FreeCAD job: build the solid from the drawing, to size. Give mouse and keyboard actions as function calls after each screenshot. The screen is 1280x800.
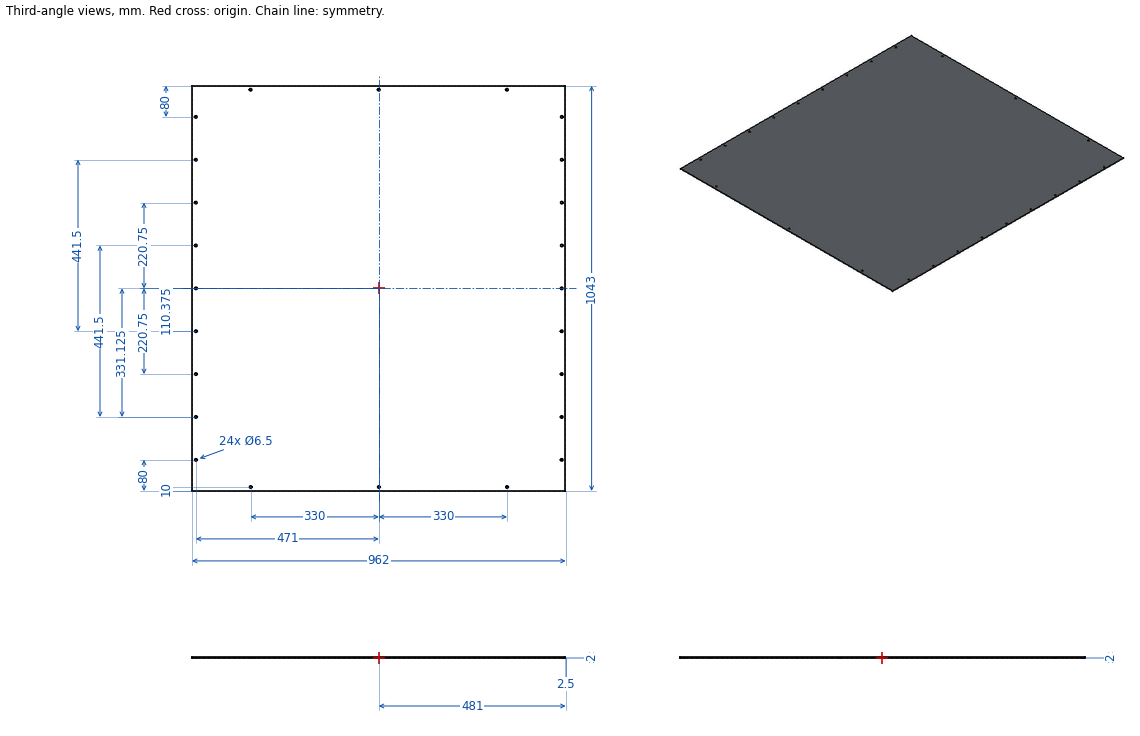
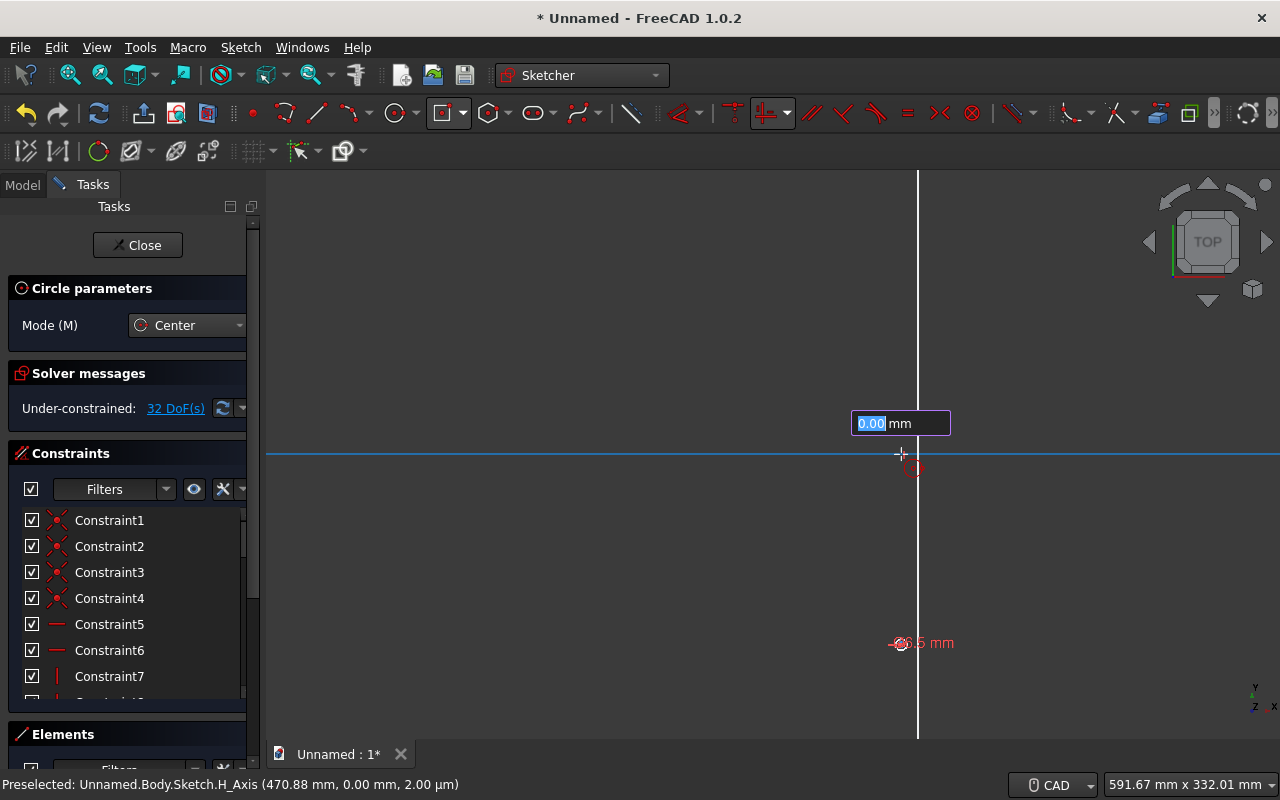
scroll(899, 460, up, 6)
move(899, 458)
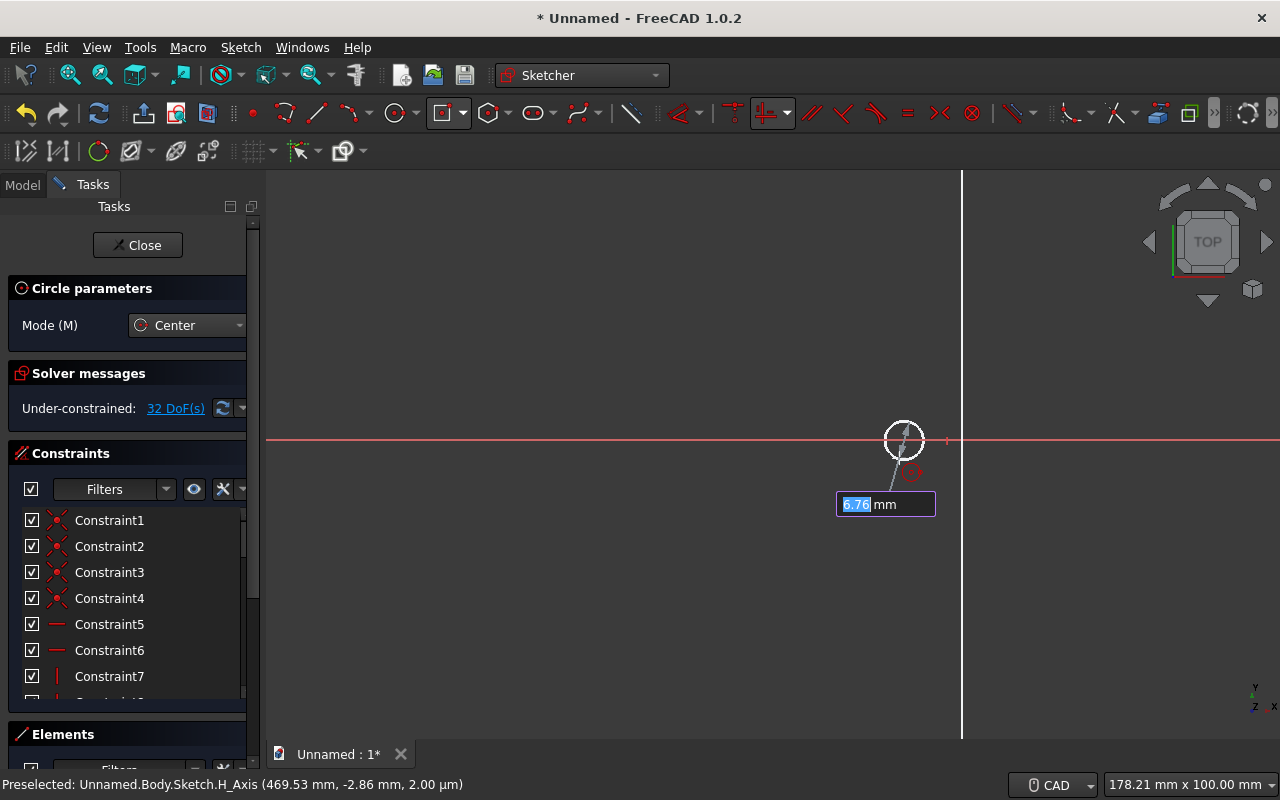
text(6.5)
key(Return)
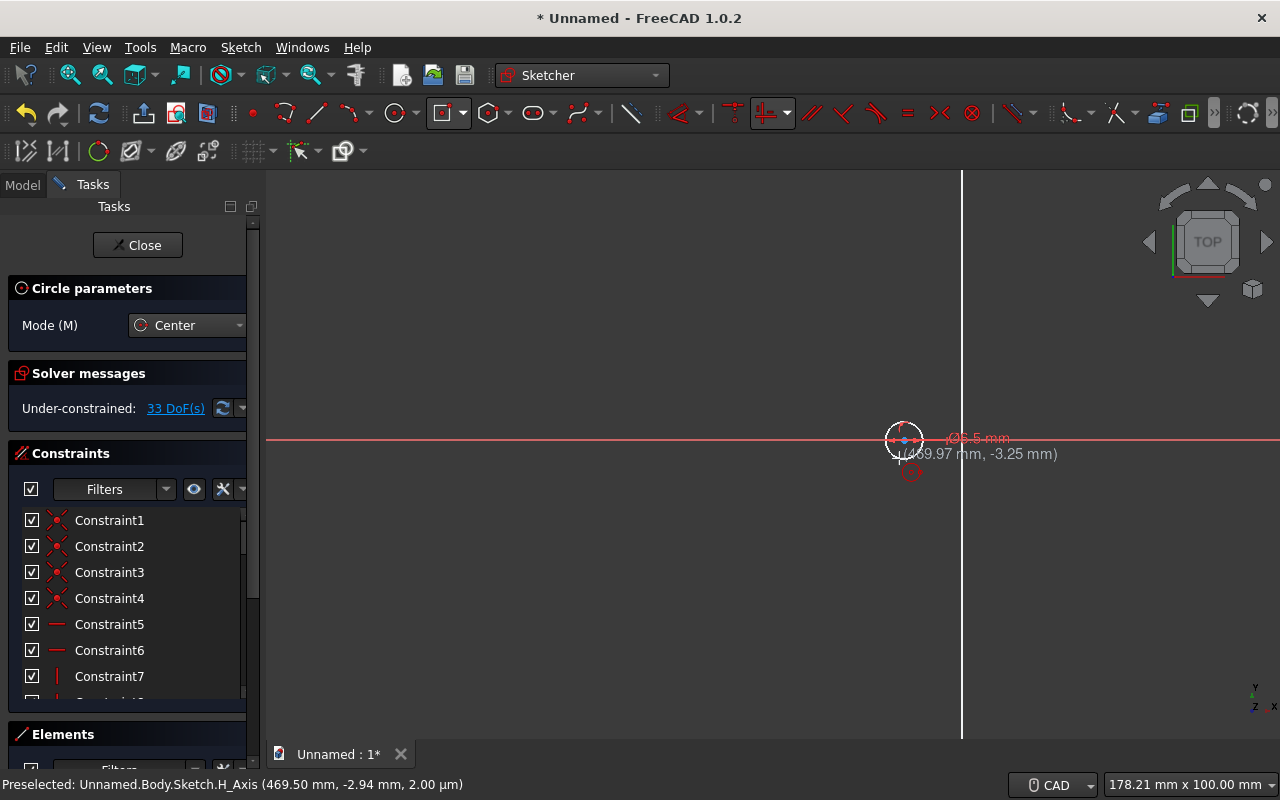
scroll(865, 455, down, 14)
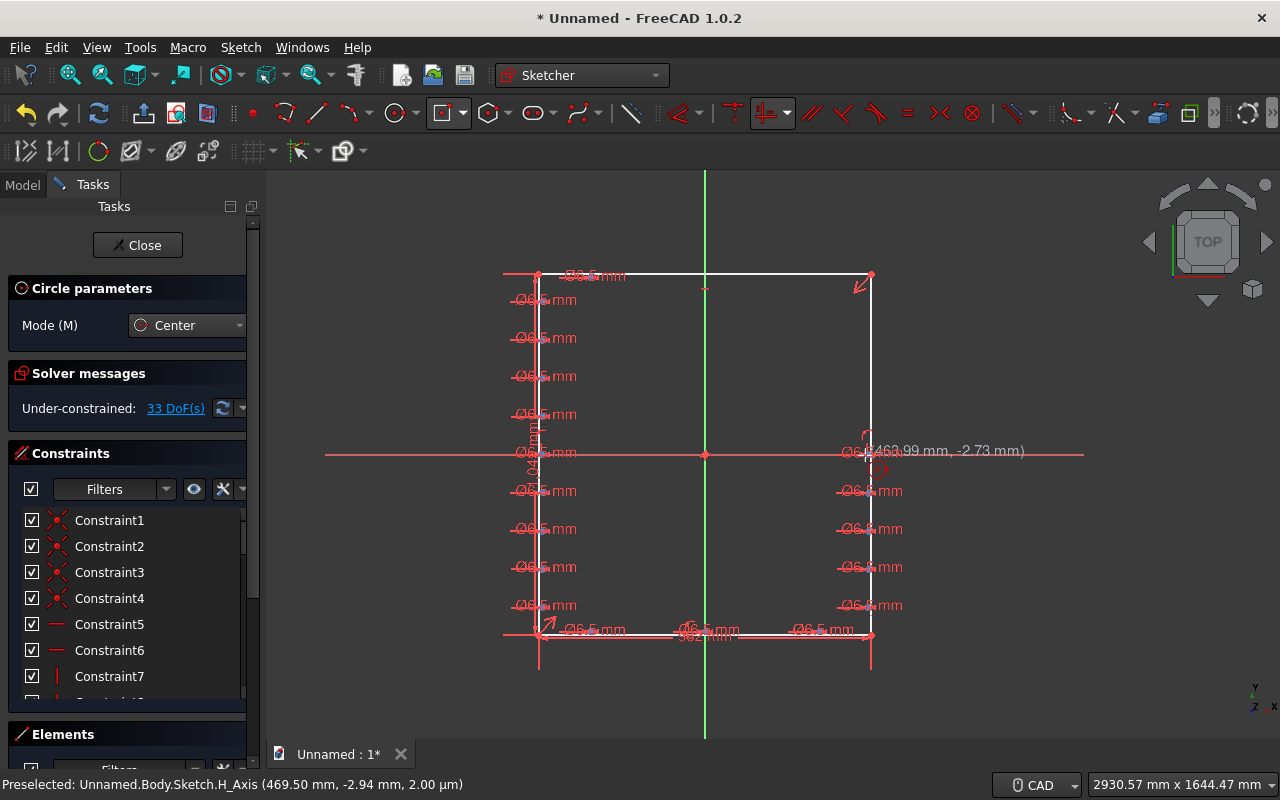
scroll(868, 416, up, 16)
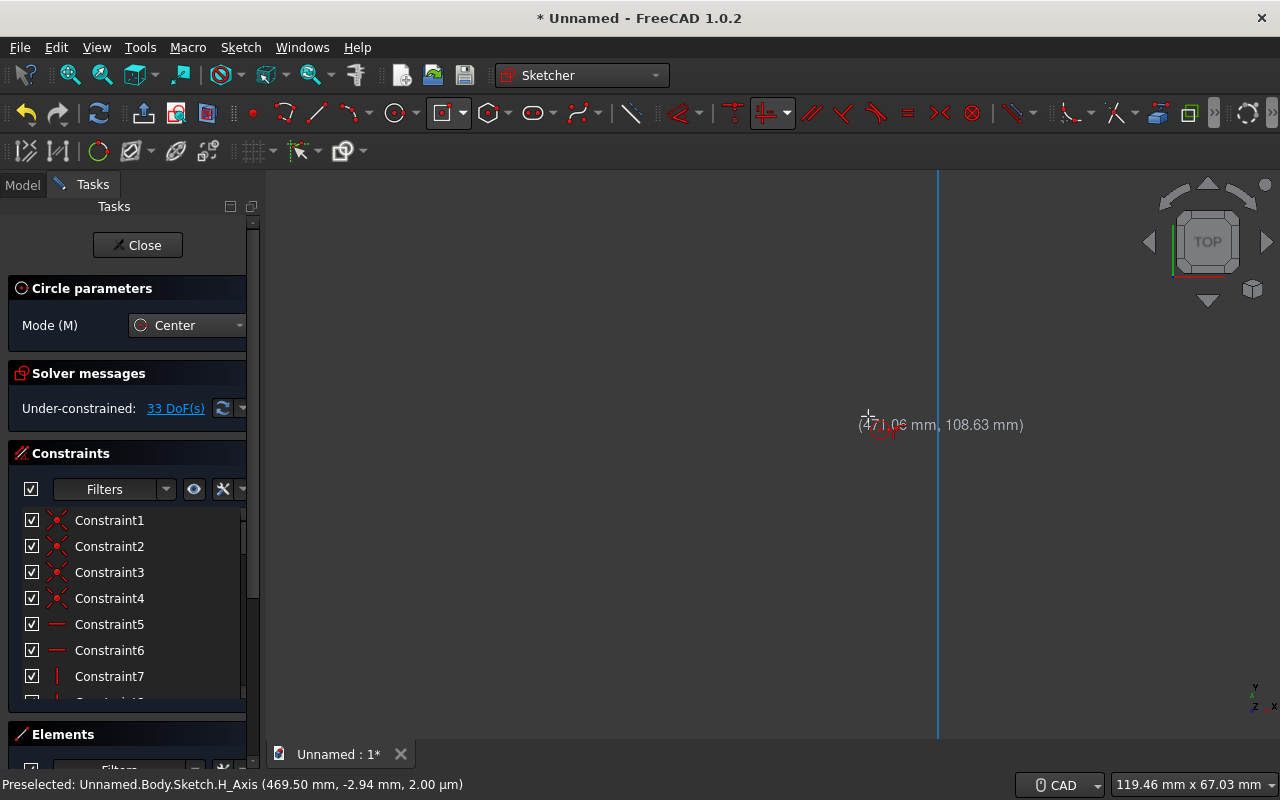
scroll(906, 407, down, 15)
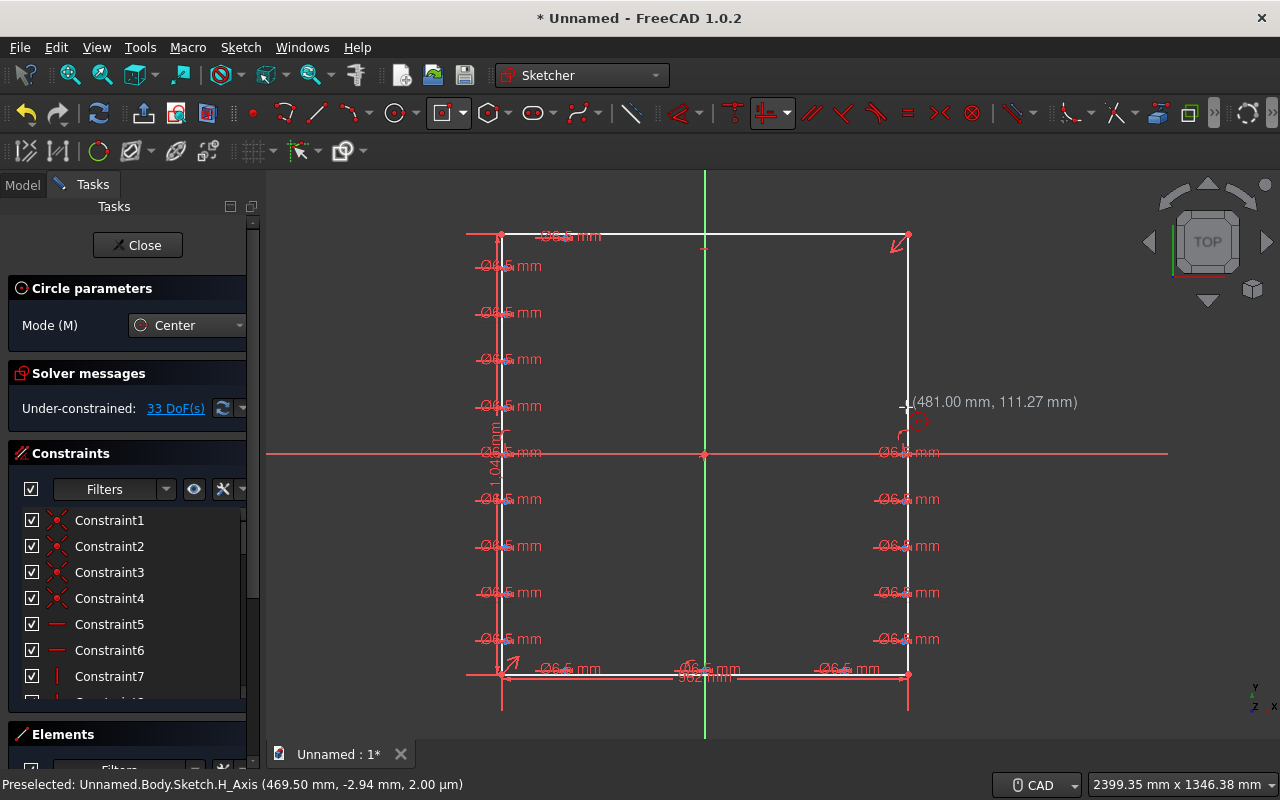
scroll(904, 408, up, 7)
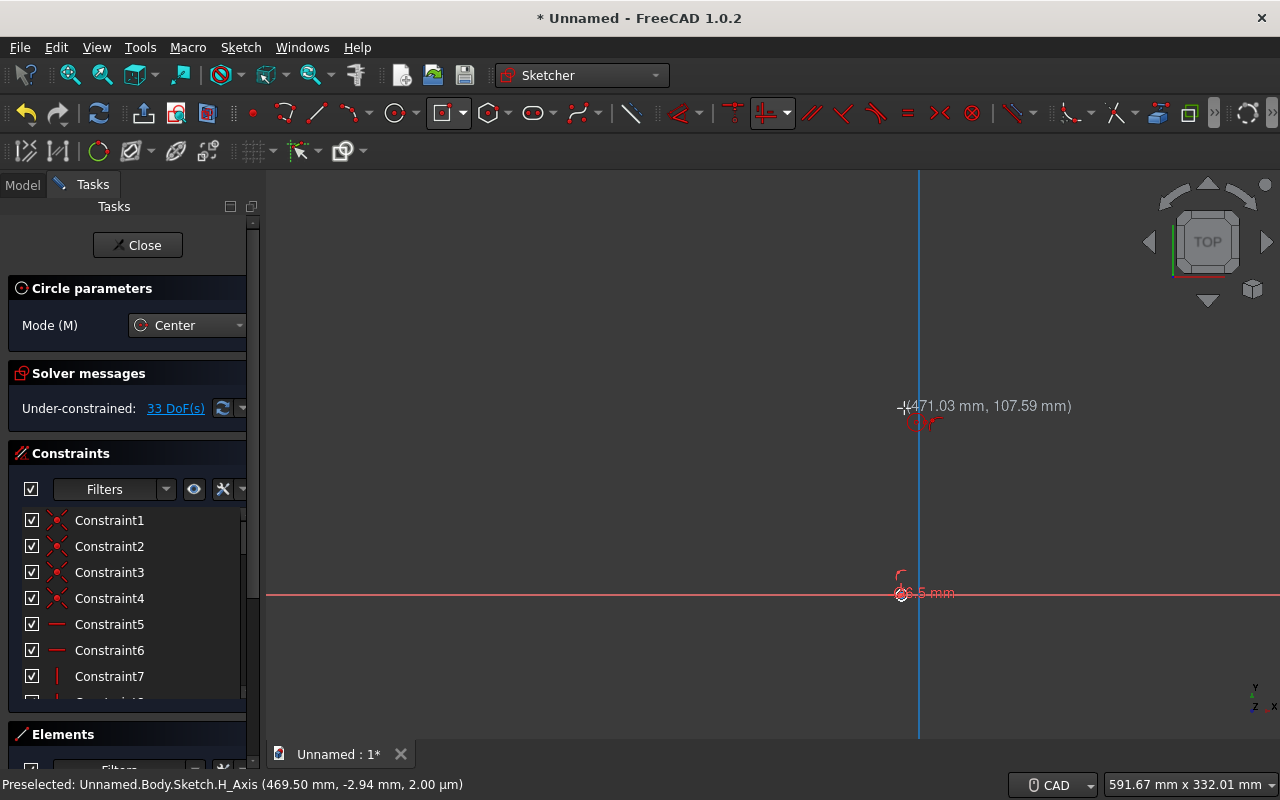
click(902, 406)
move(898, 402)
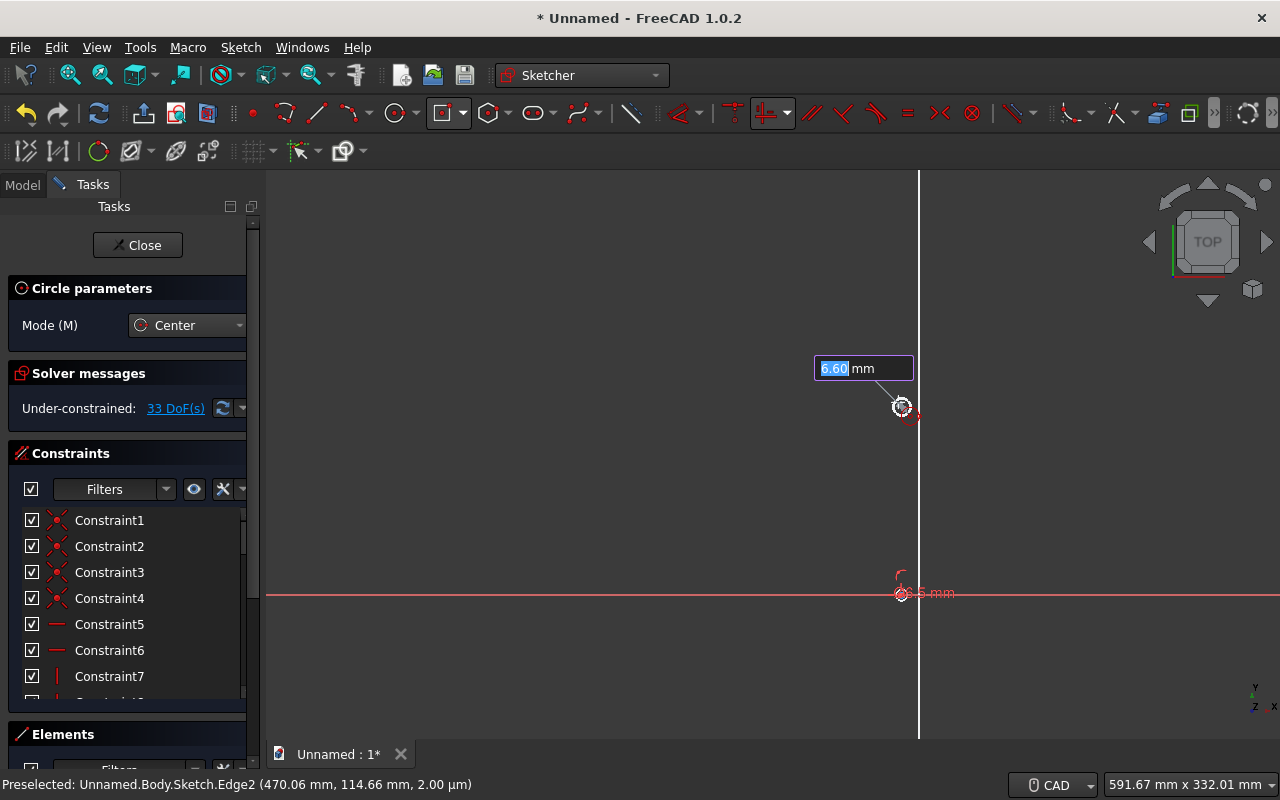
text(6.5)
key(Return)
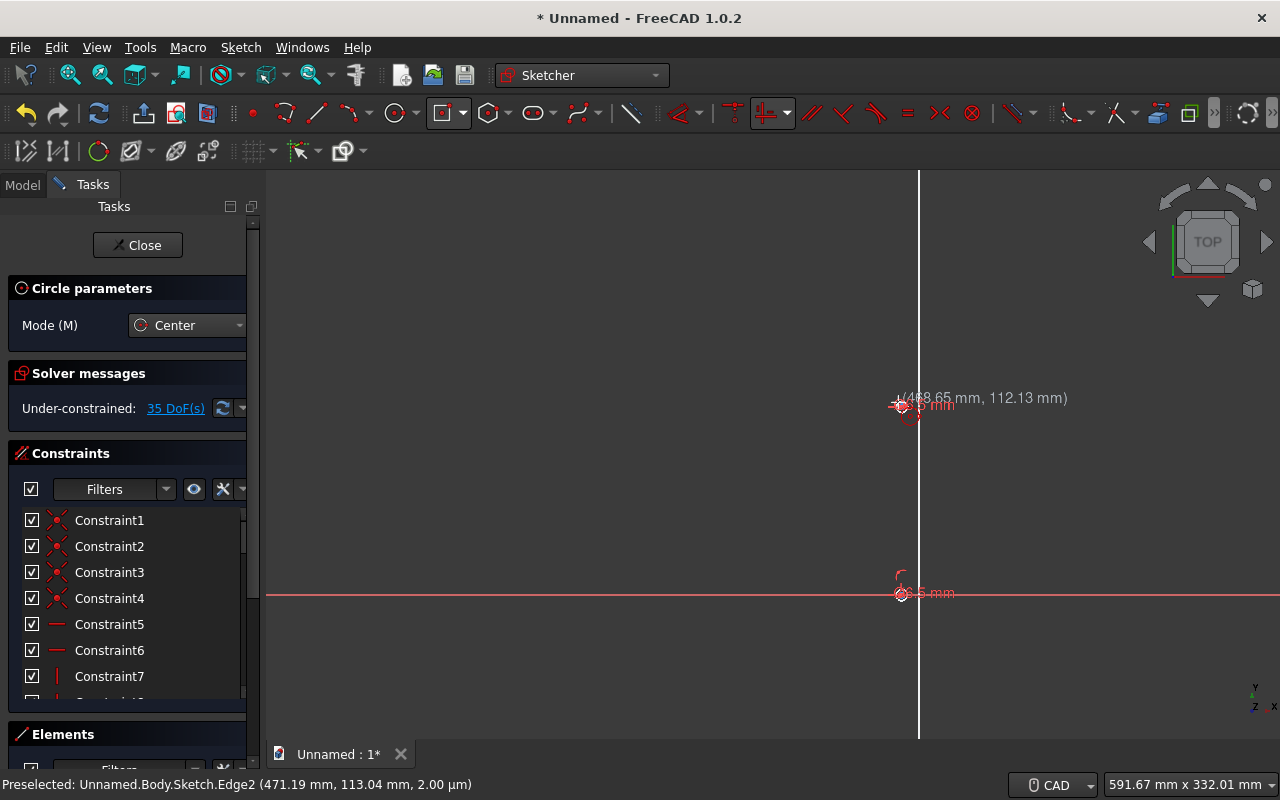
scroll(902, 217, up, 8)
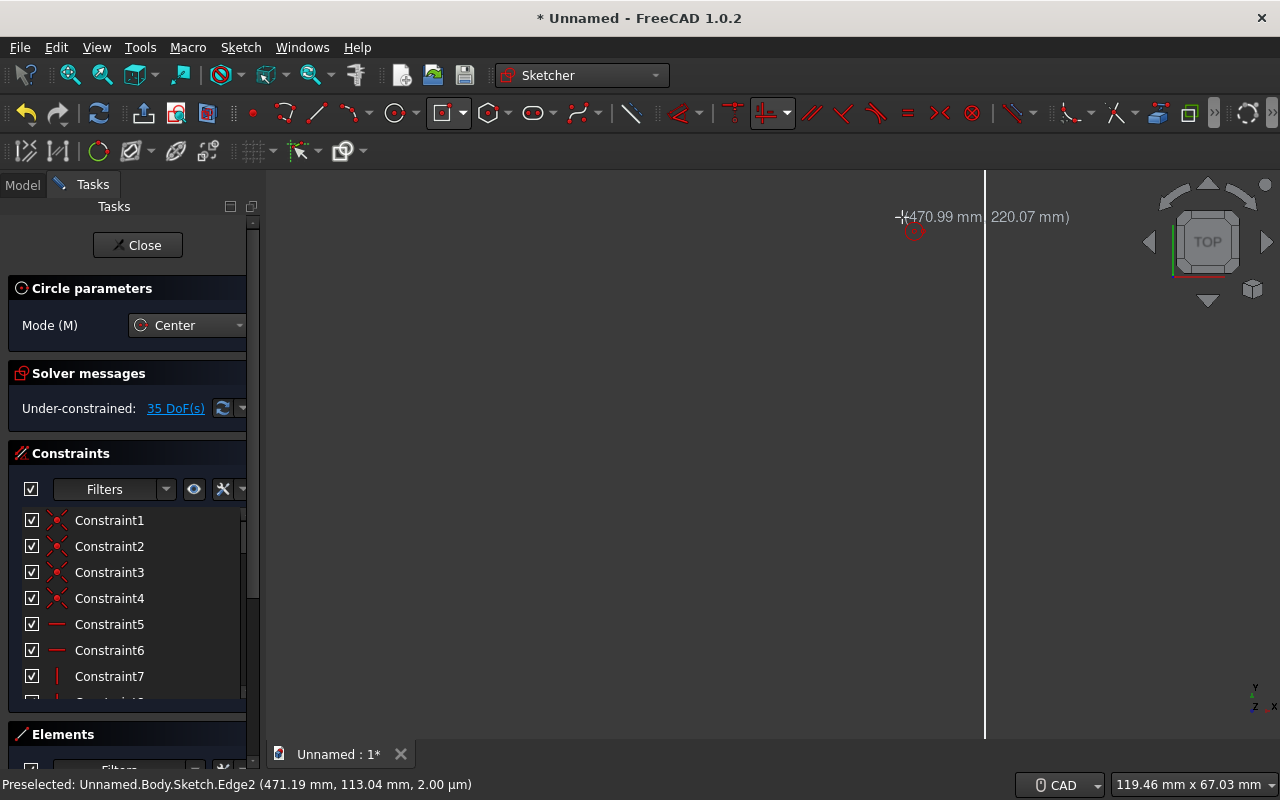
scroll(904, 369, down, 15)